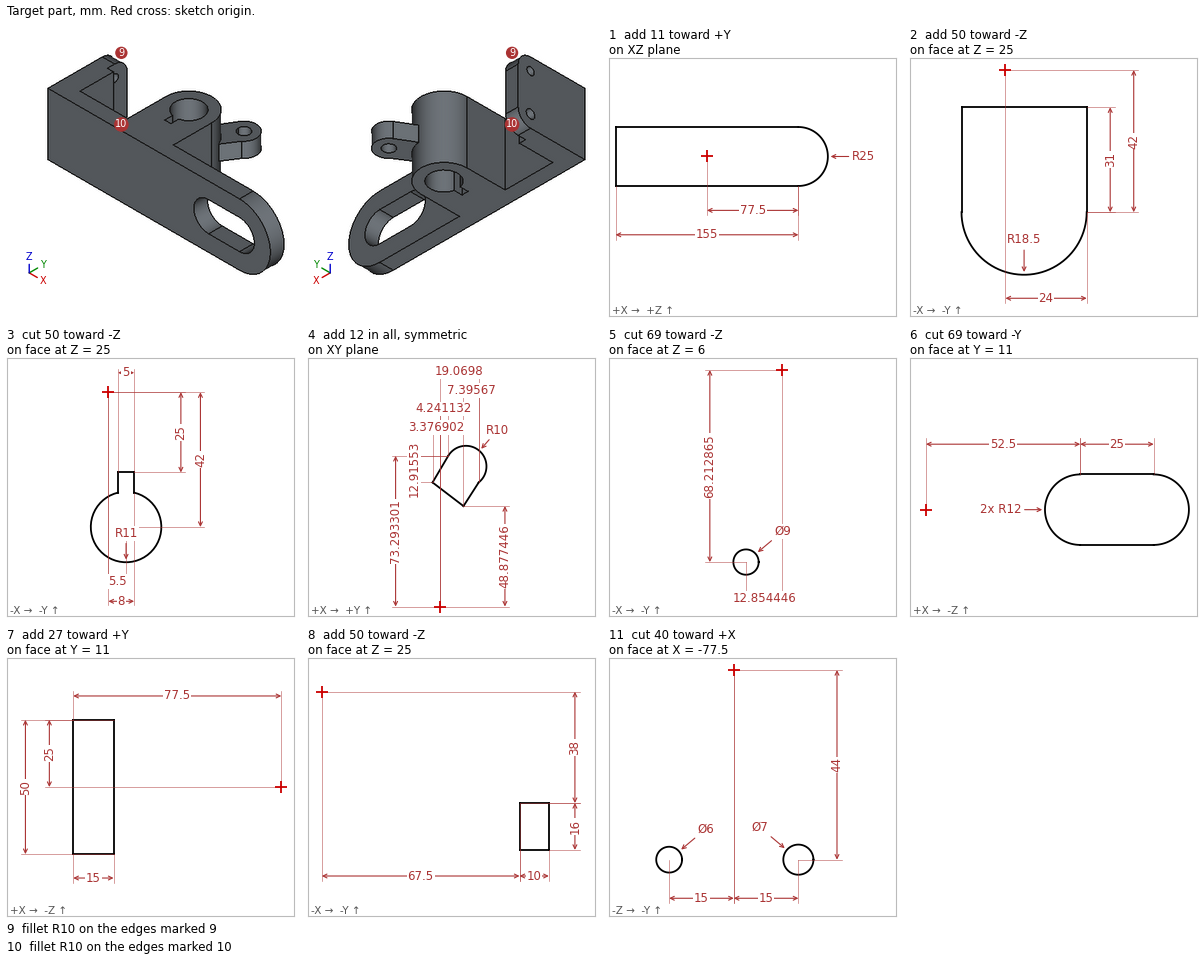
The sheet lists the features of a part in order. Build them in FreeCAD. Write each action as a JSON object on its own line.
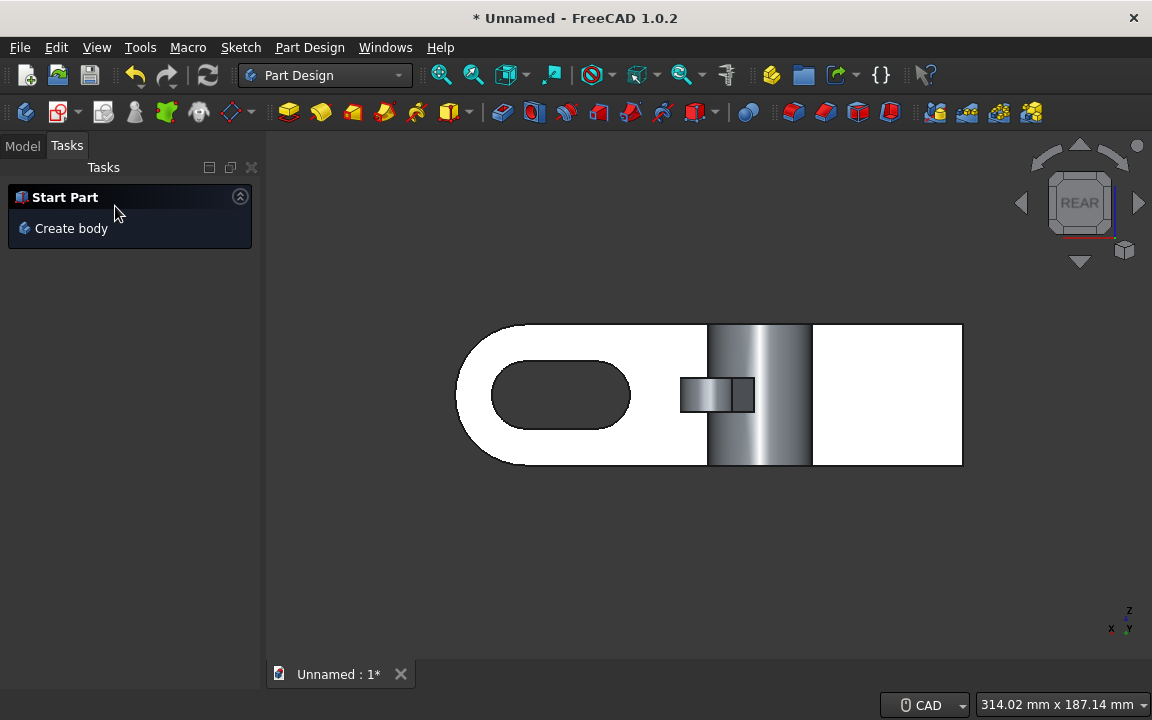
{"action": "left_click", "coordinate": [653, 354]}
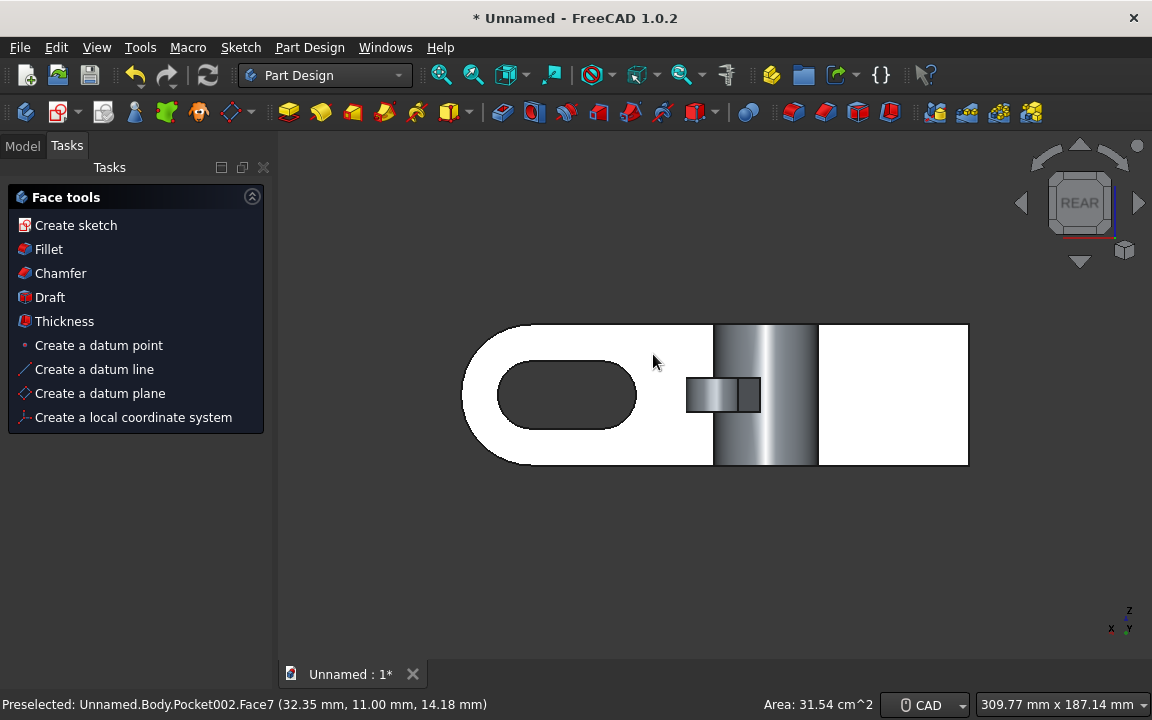
{"action": "left_click", "coordinate": [58, 112]}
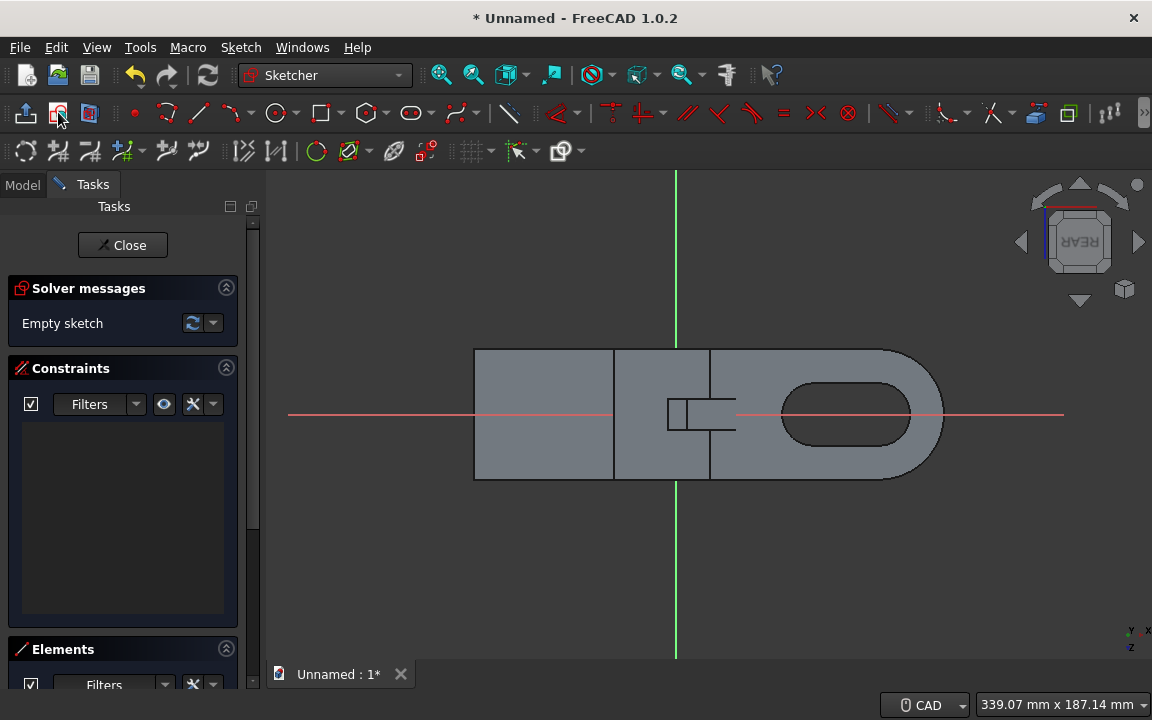
{"action": "left_click", "coordinate": [90, 114]}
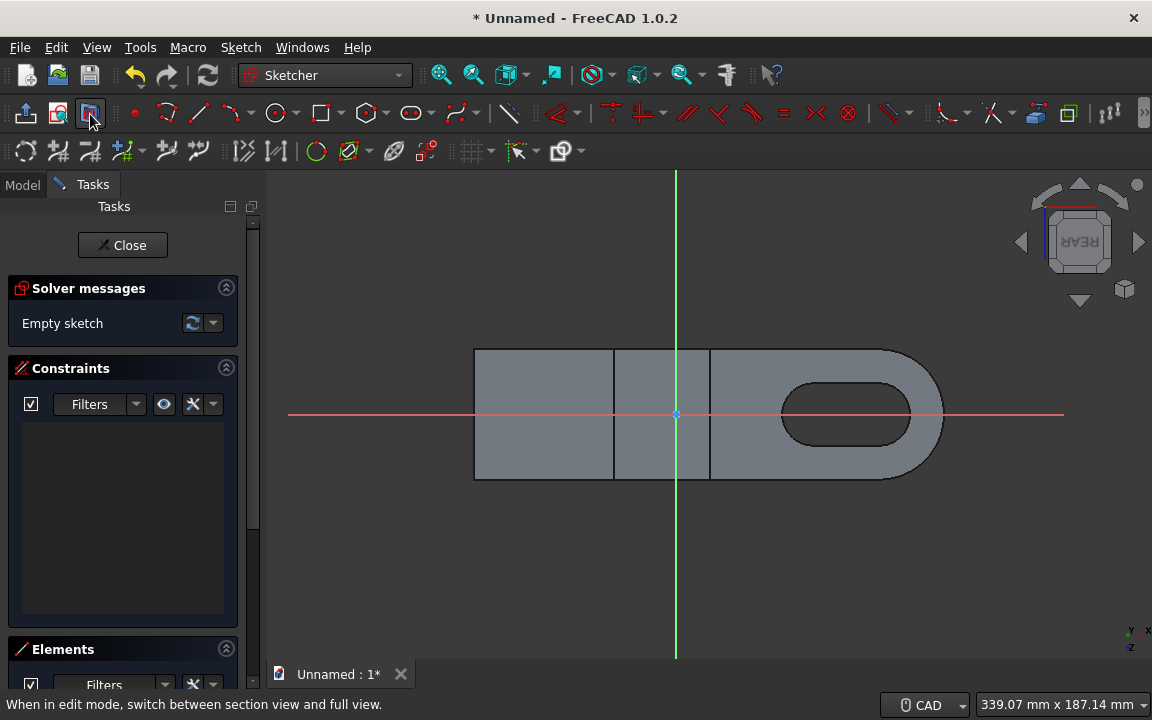
{"action": "scroll", "coordinate": [522, 414], "scroll_direction": "up", "scroll_amount": 4}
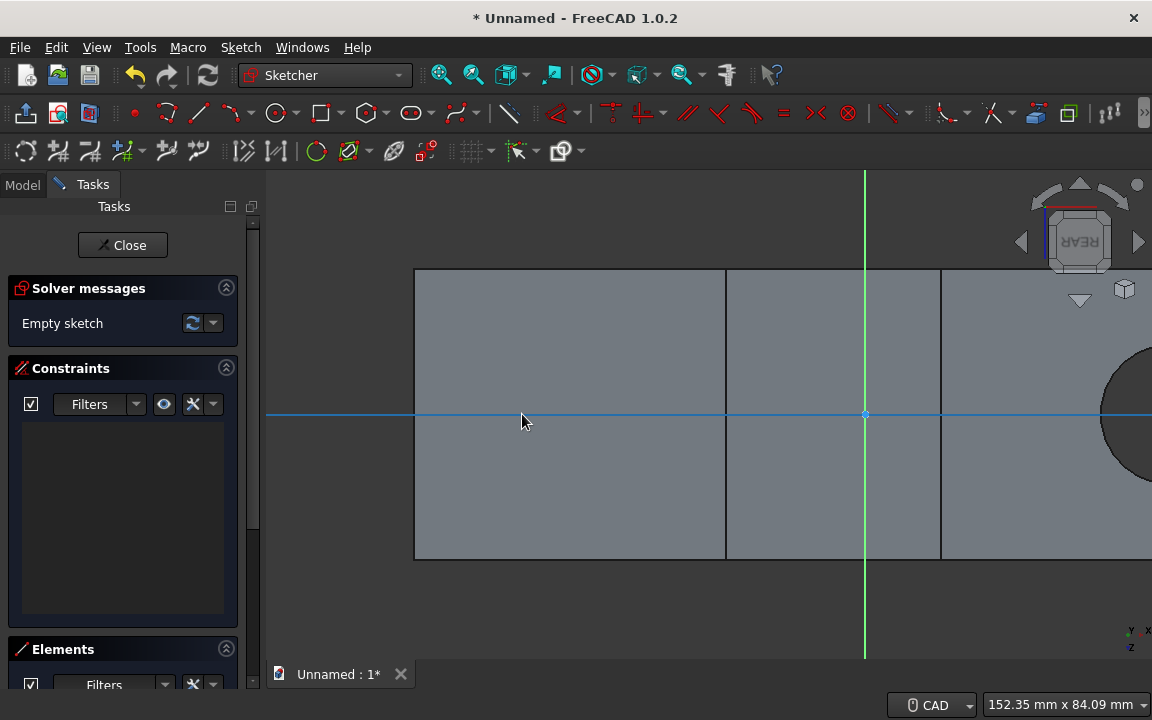
{"action": "left_click", "coordinate": [322, 114]}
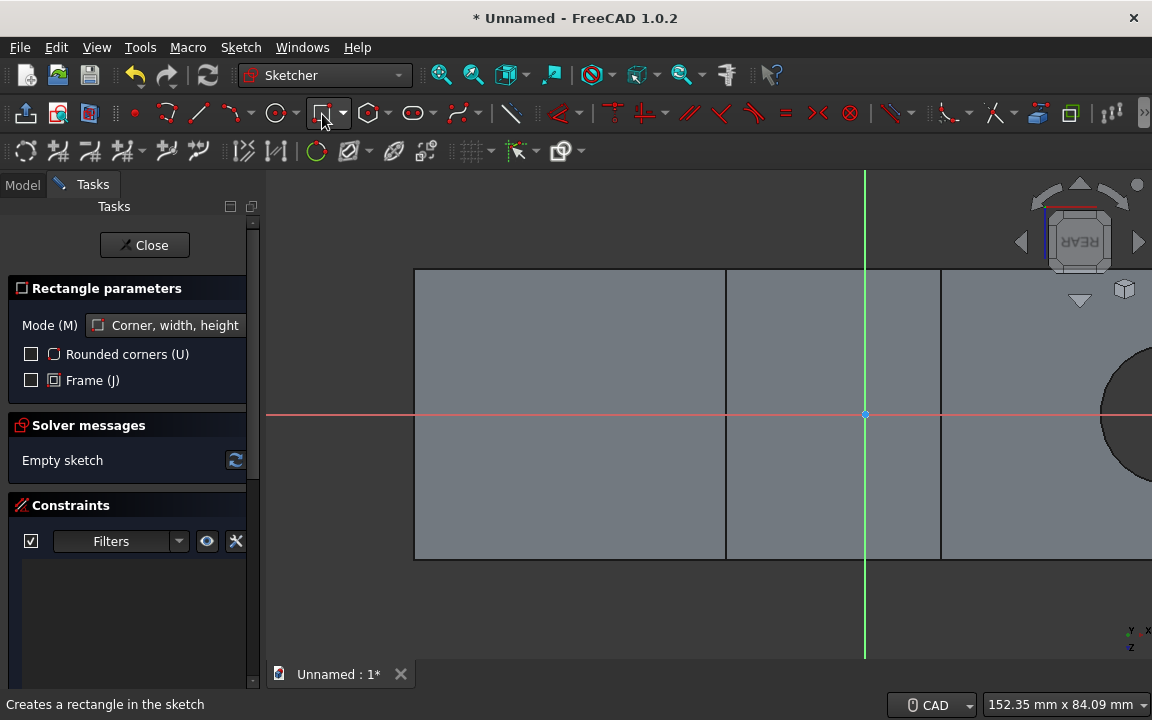
{"action": "left_click", "coordinate": [414, 269]}
{"action": "mouse_move", "coordinate": [502, 560]}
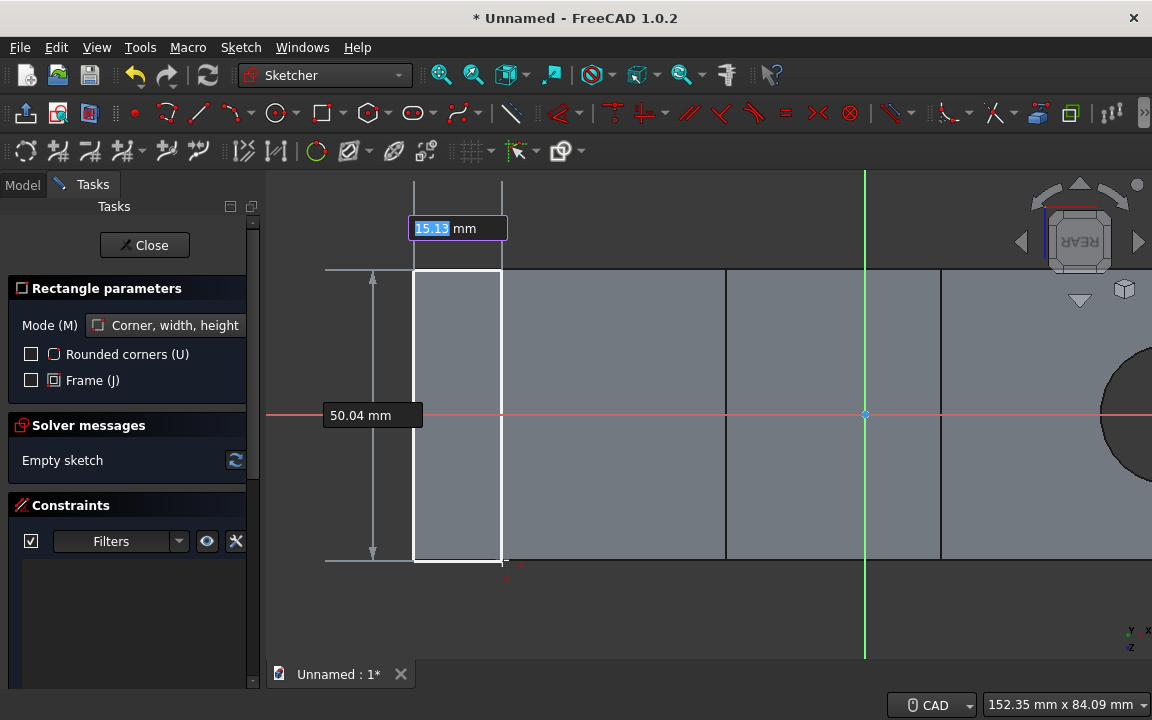
{"action": "type", "text": "15"}
{"action": "key", "text": "Tab"}
{"action": "type", "text": "50"}
{"action": "key", "text": "Return"}
{"action": "key", "text": "Escape"}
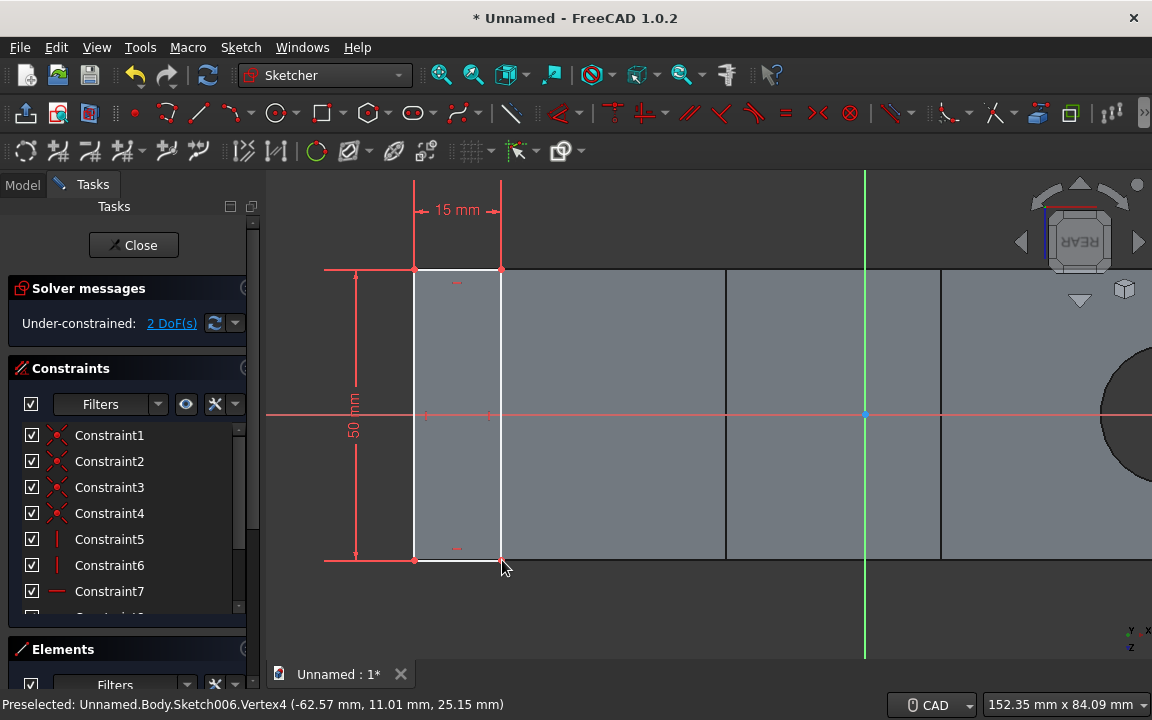
{"action": "left_click", "coordinate": [558, 114]}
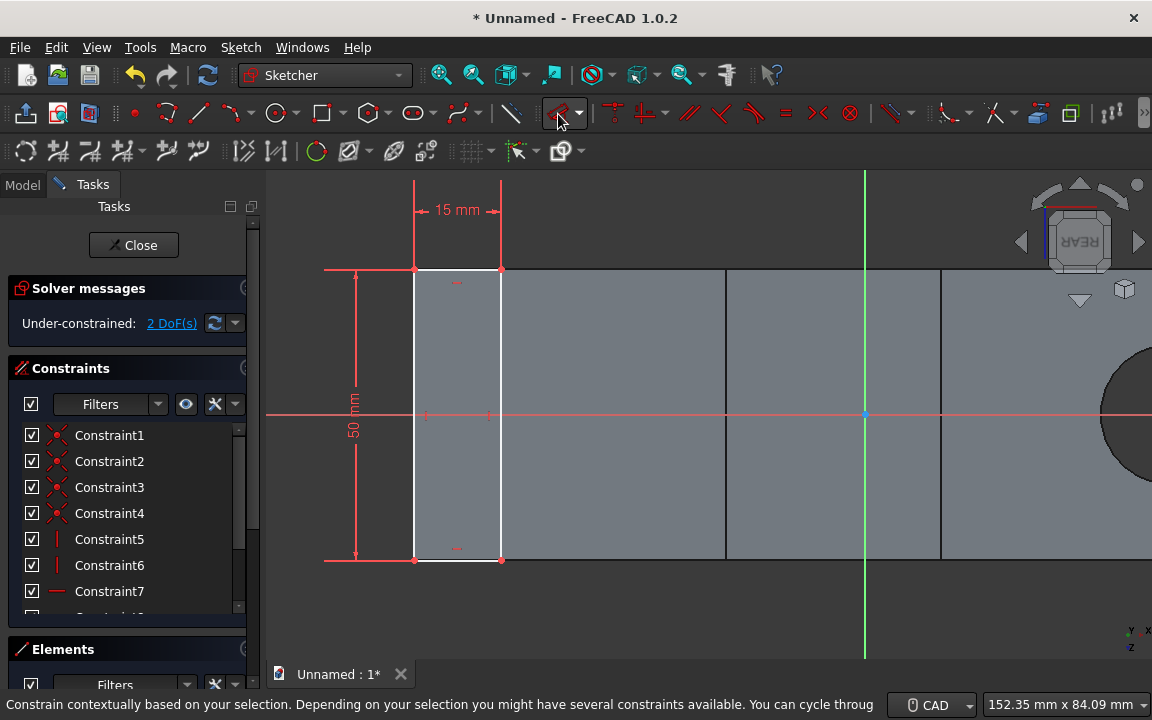
{"action": "left_click", "coordinate": [414, 270]}
{"action": "left_click", "coordinate": [380, 342]}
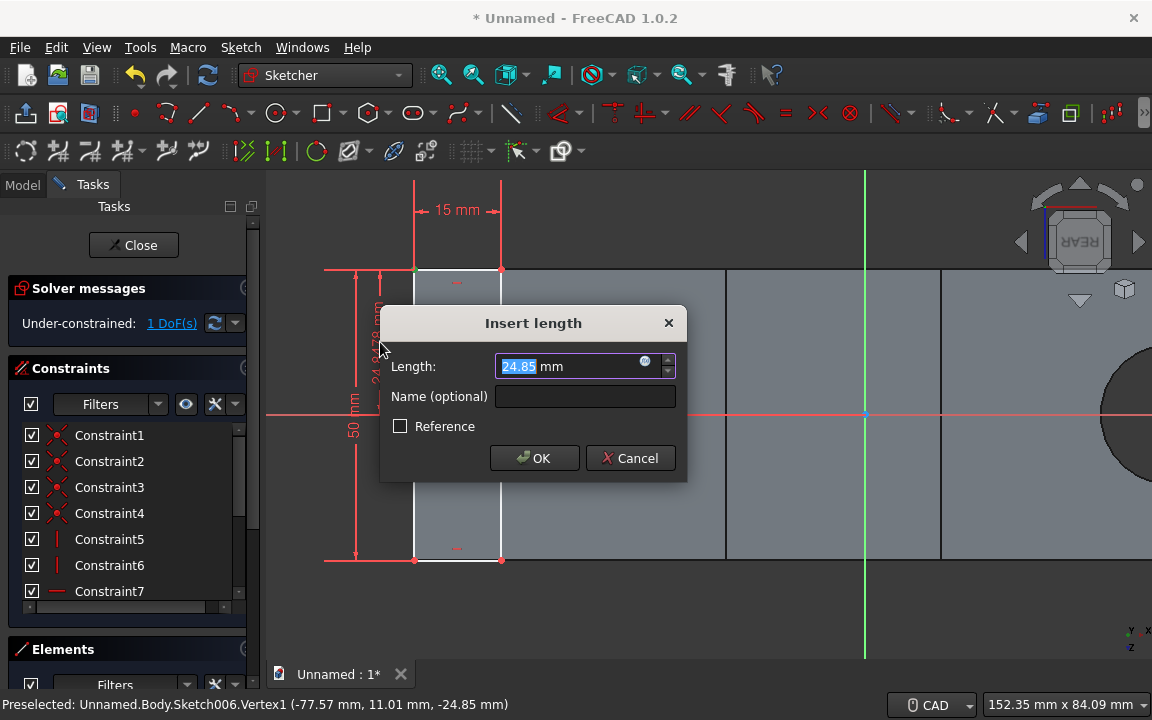
{"action": "type", "text": "25"}
{"action": "key", "text": "Return"}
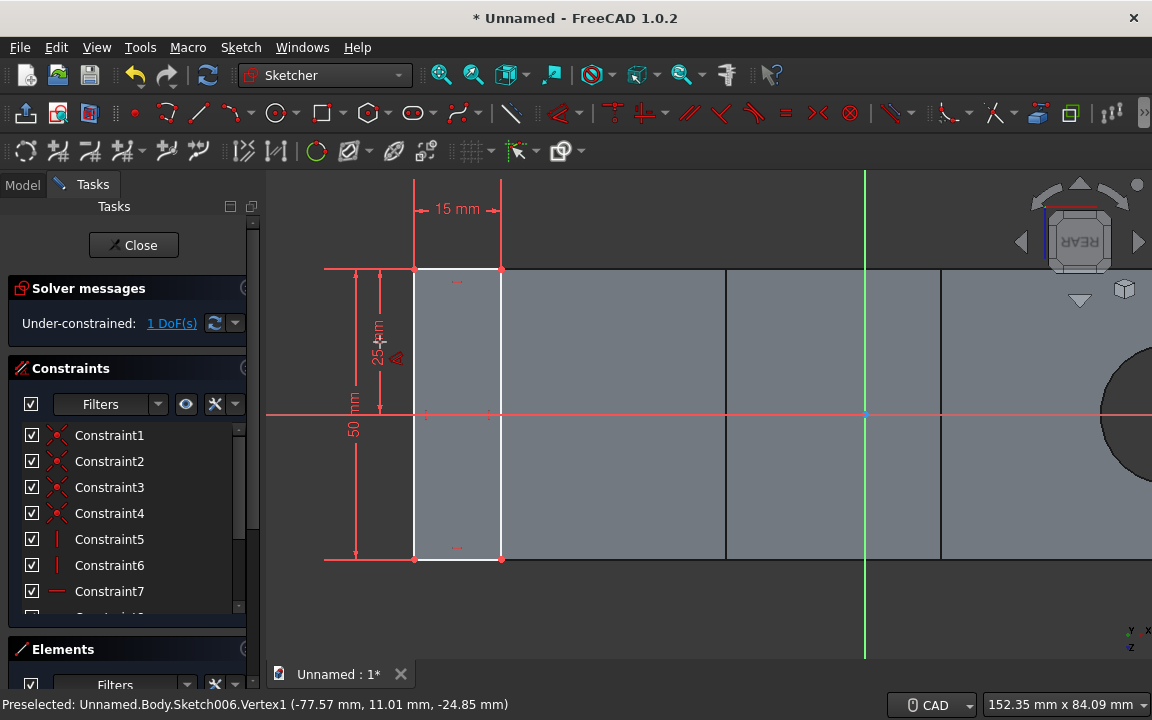
{"action": "left_click", "coordinate": [414, 269]}
{"action": "left_click", "coordinate": [640, 235]}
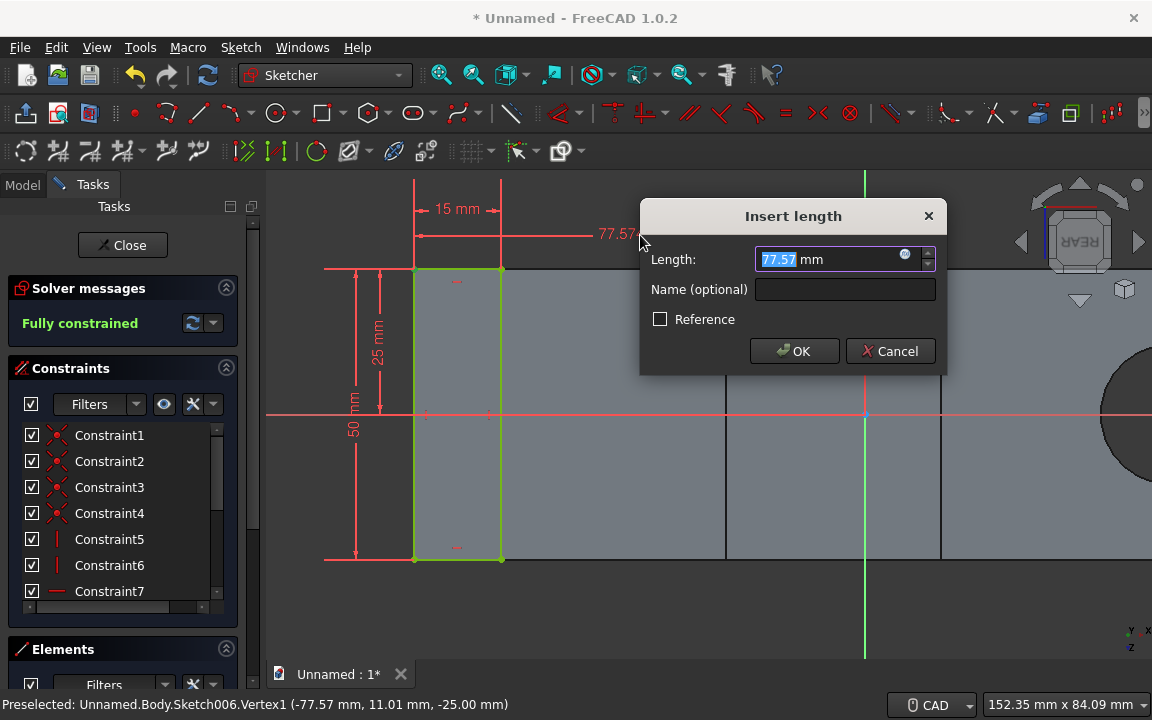
{"action": "type", "text": "77.5"}
{"action": "key", "text": "Return"}
{"action": "key", "text": "Escape"}